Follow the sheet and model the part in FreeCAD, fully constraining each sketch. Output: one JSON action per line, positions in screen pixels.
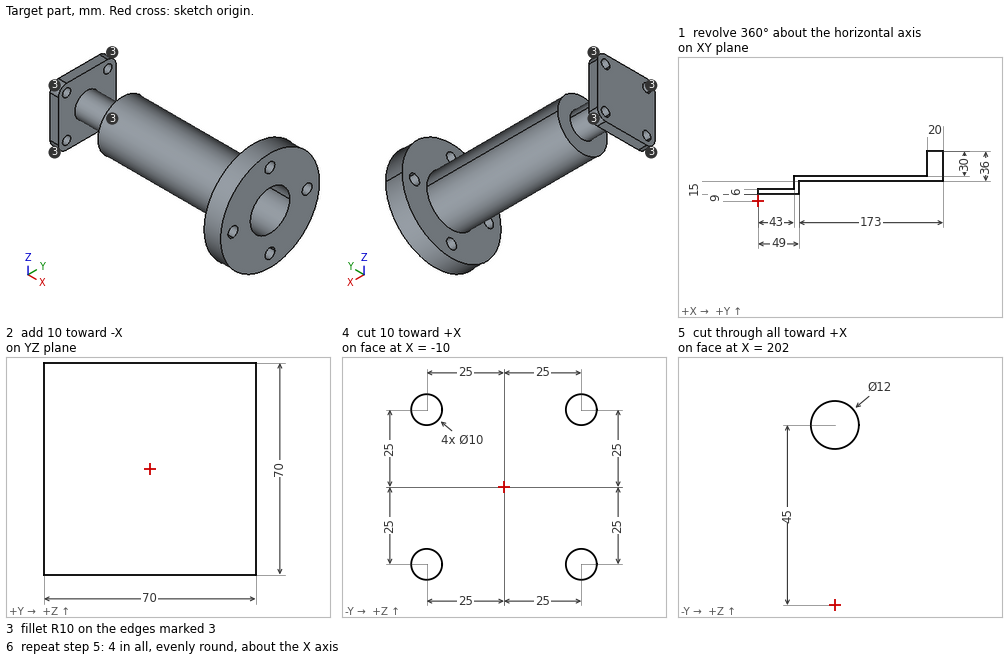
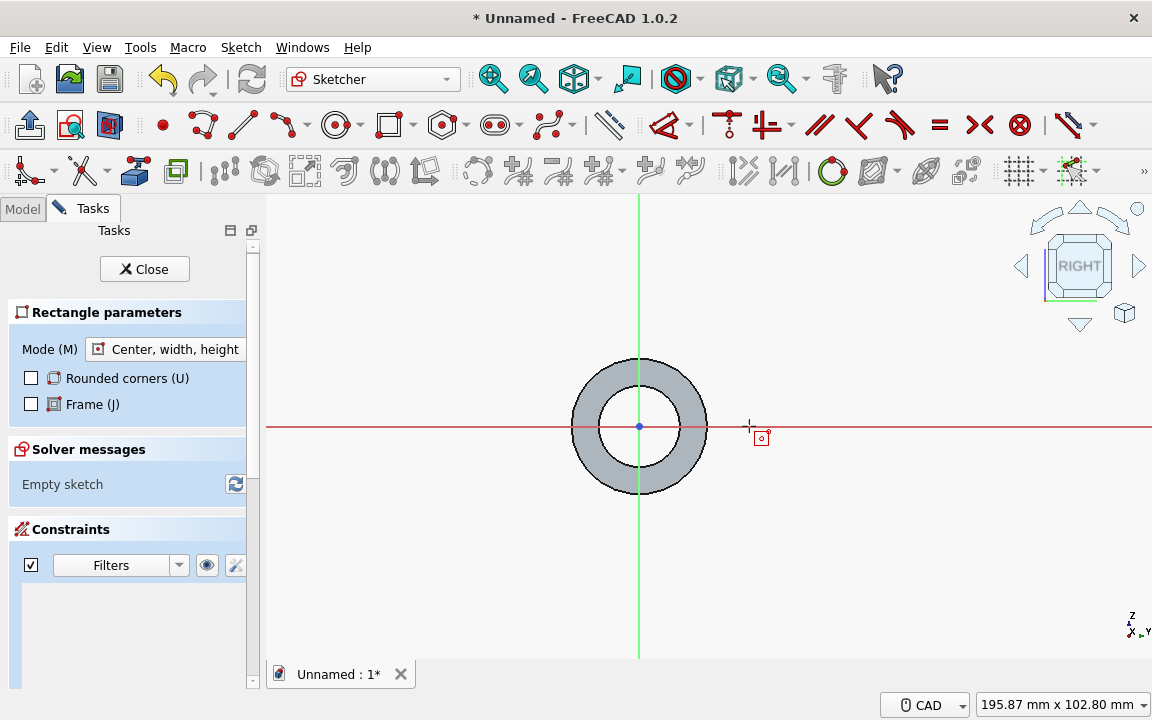
{"action": "left_click", "coordinate": [639, 426]}
{"action": "mouse_move", "coordinate": [798, 268]}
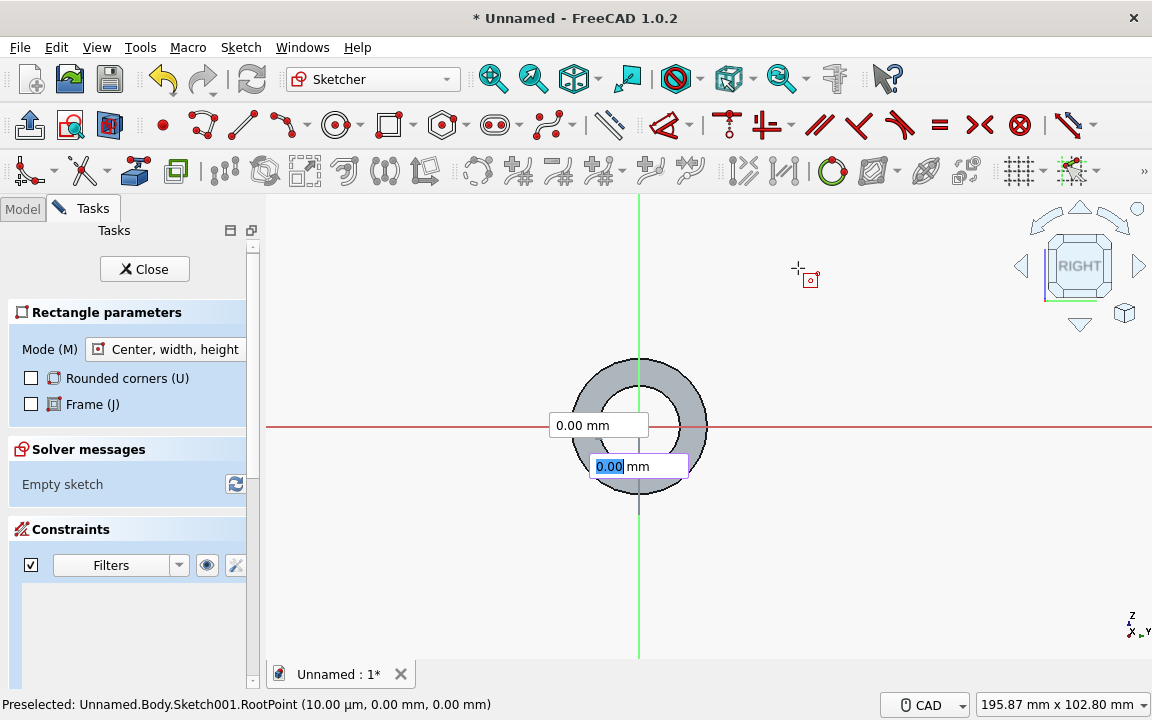
{"action": "type", "text": "70"}
{"action": "key", "text": "Tab"}
{"action": "type", "text": "70"}
{"action": "key", "text": "Return"}
{"action": "key", "text": "Escape"}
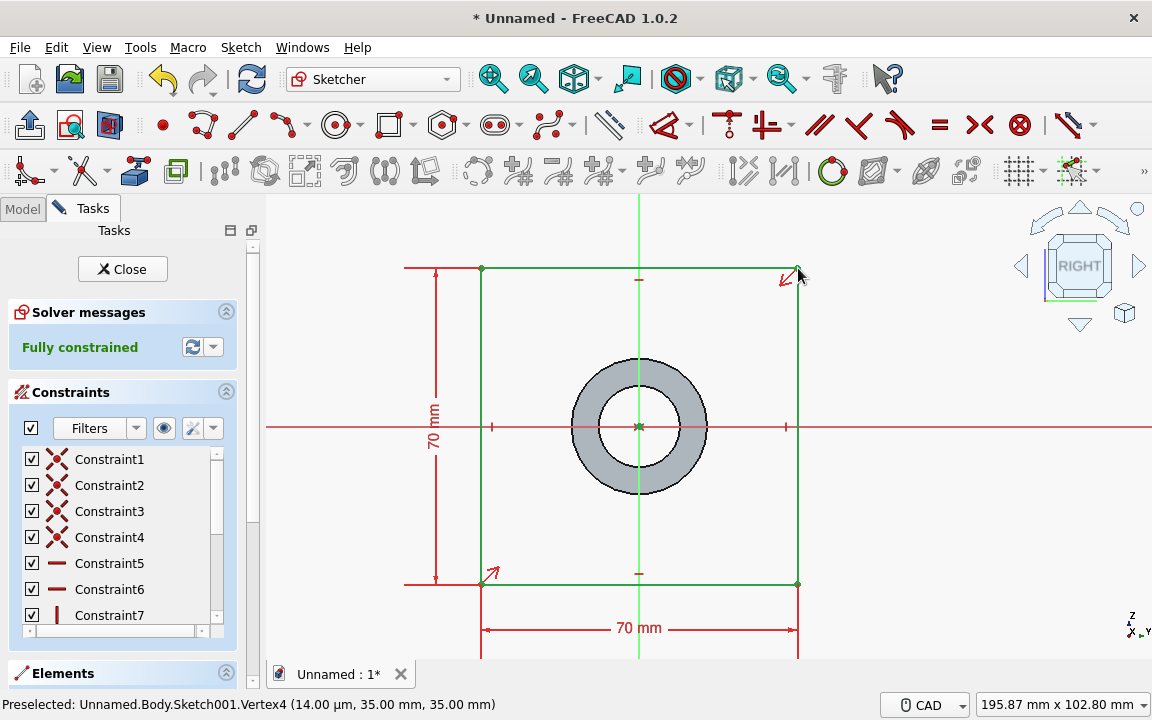
{"action": "left_click", "coordinate": [123, 269]}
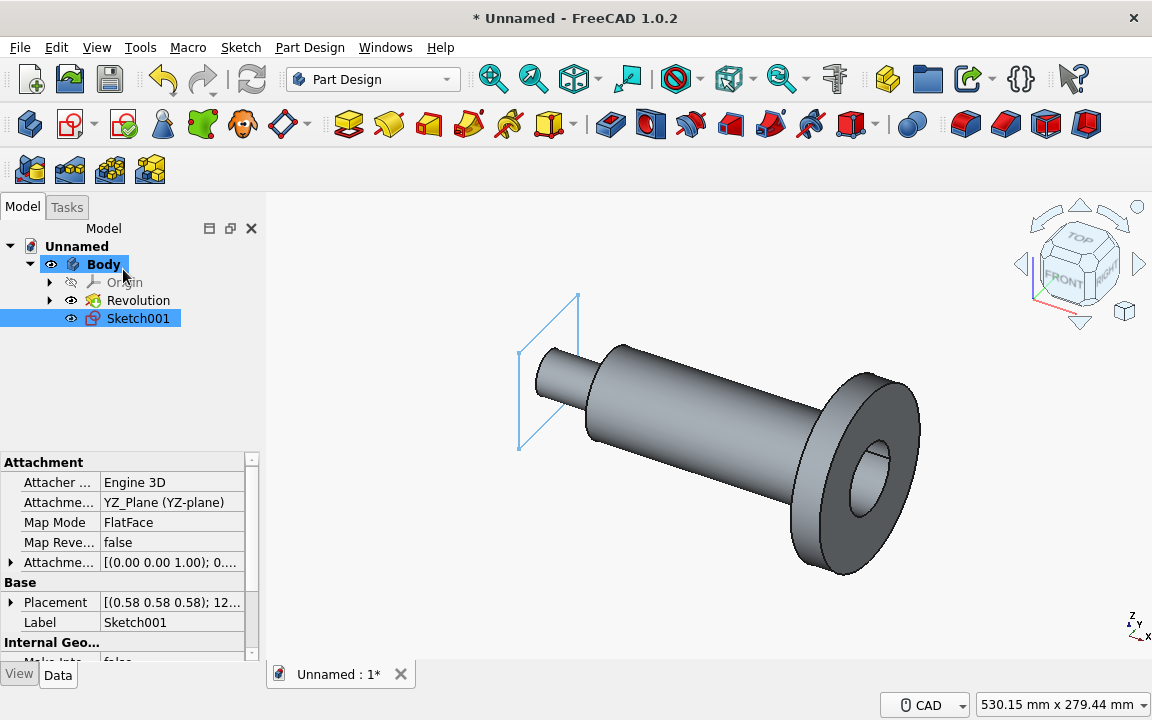
{"action": "left_click", "coordinate": [350, 124]}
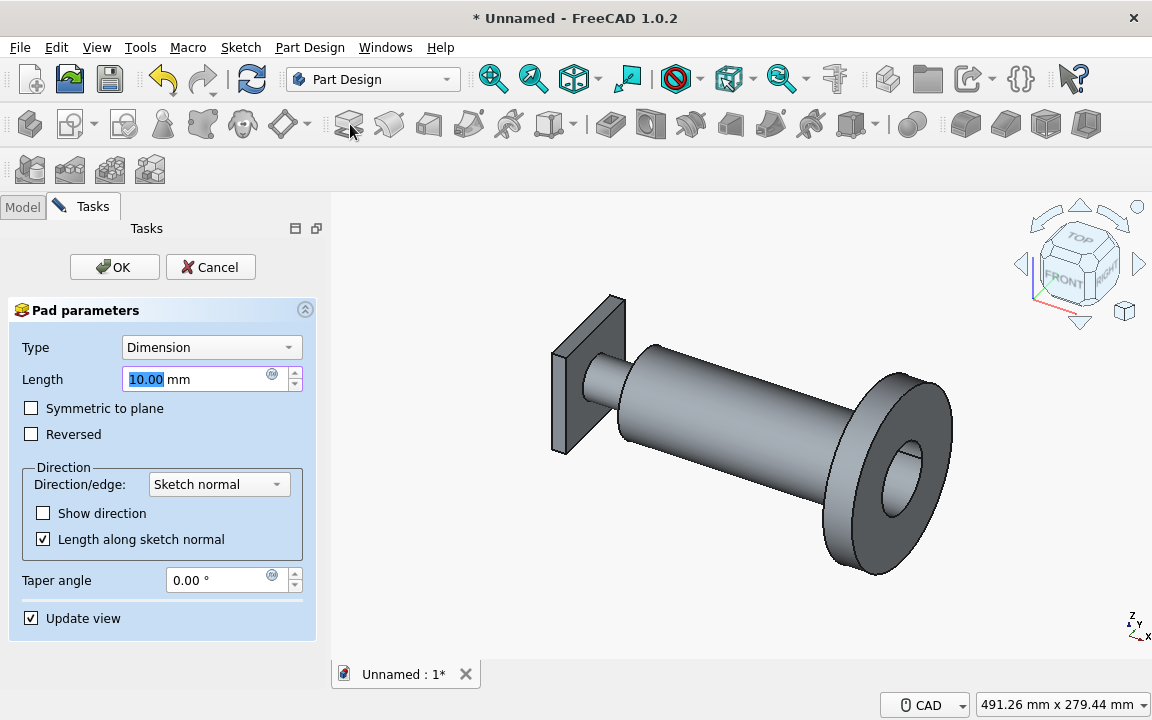
{"action": "type", "text": "10"}
{"action": "key", "text": "Tab"}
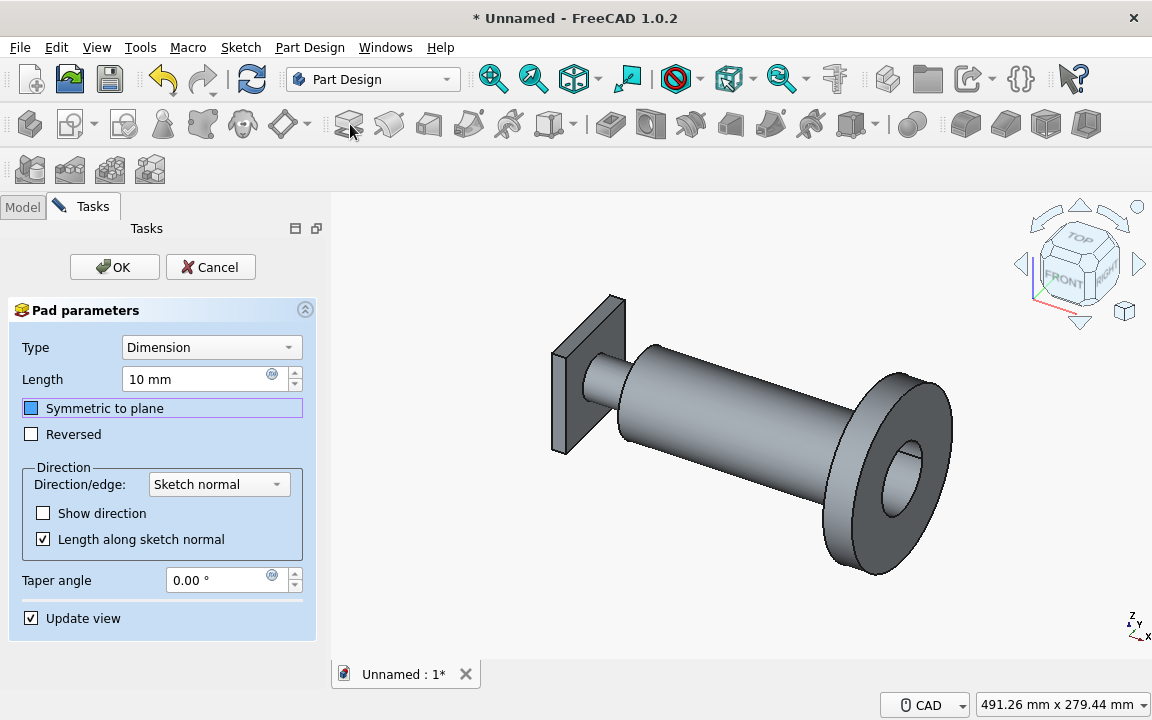
{"action": "left_click", "coordinate": [30, 434]}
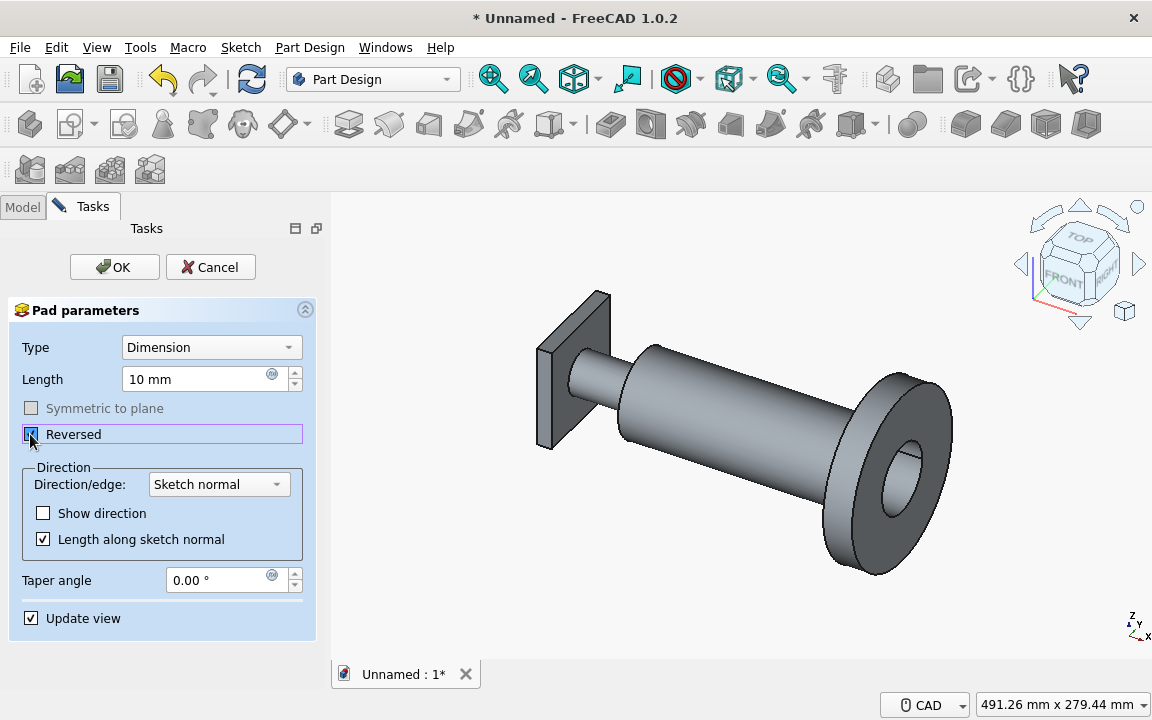
{"action": "left_click", "coordinate": [115, 267]}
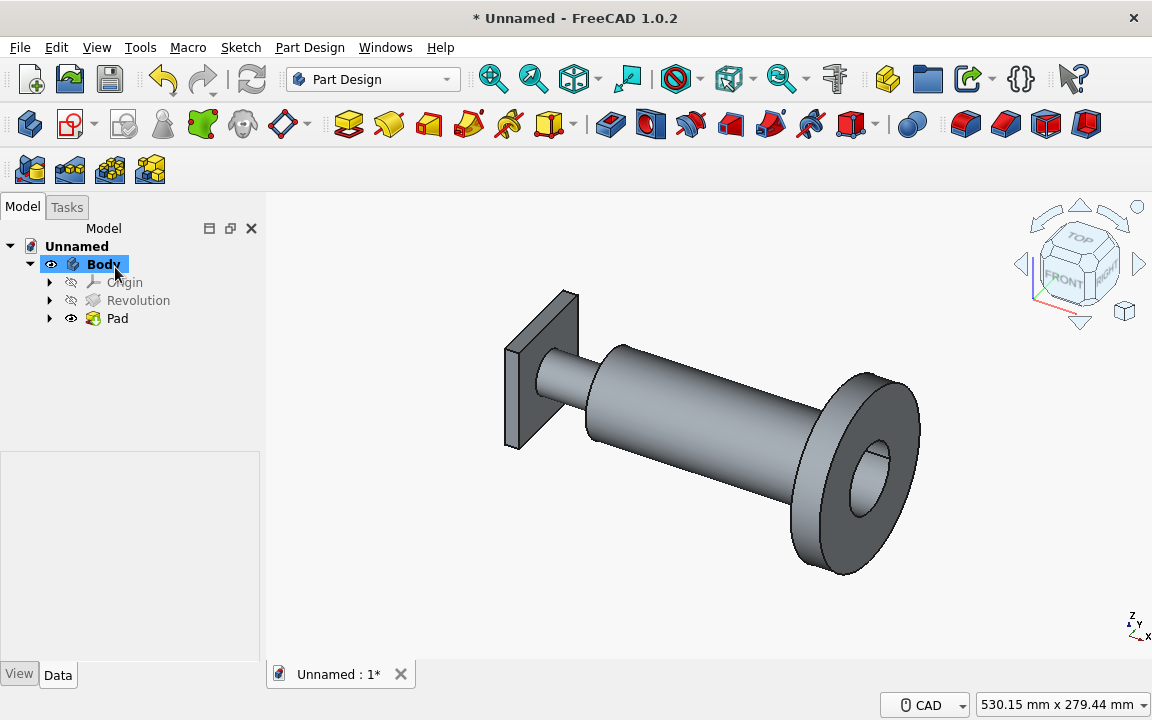
{"action": "left_click", "coordinate": [512, 350]}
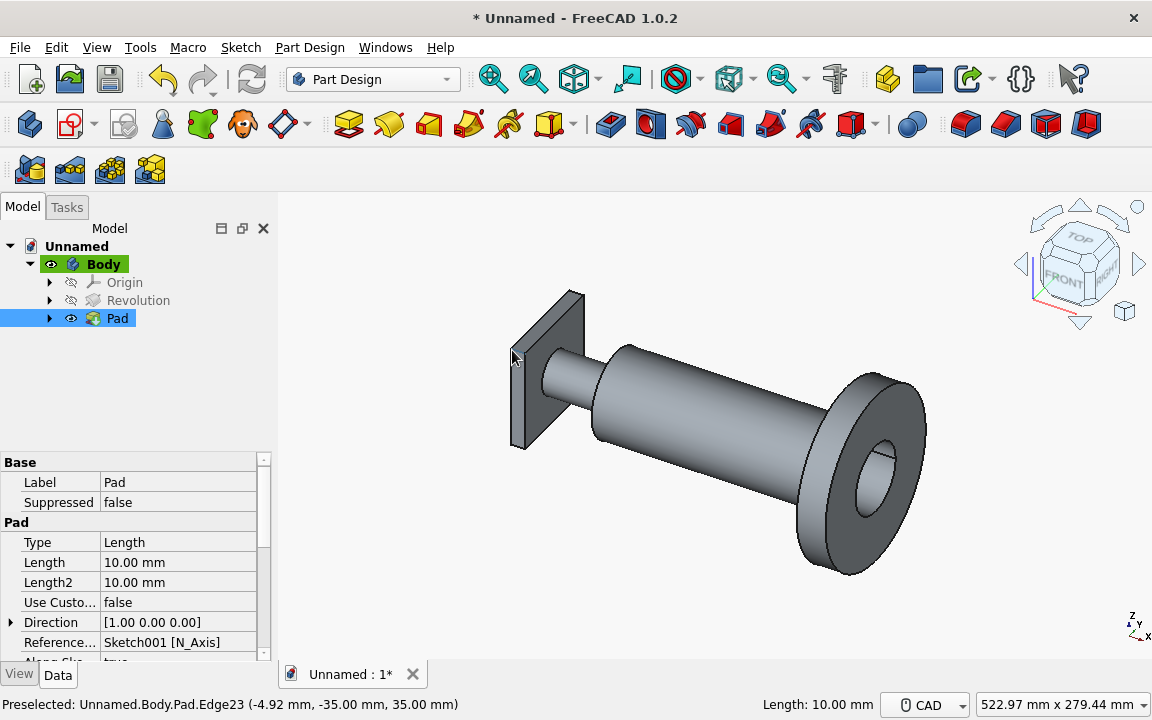
{"action": "scroll", "coordinate": [576, 292], "scroll_direction": "up", "scroll_amount": 5}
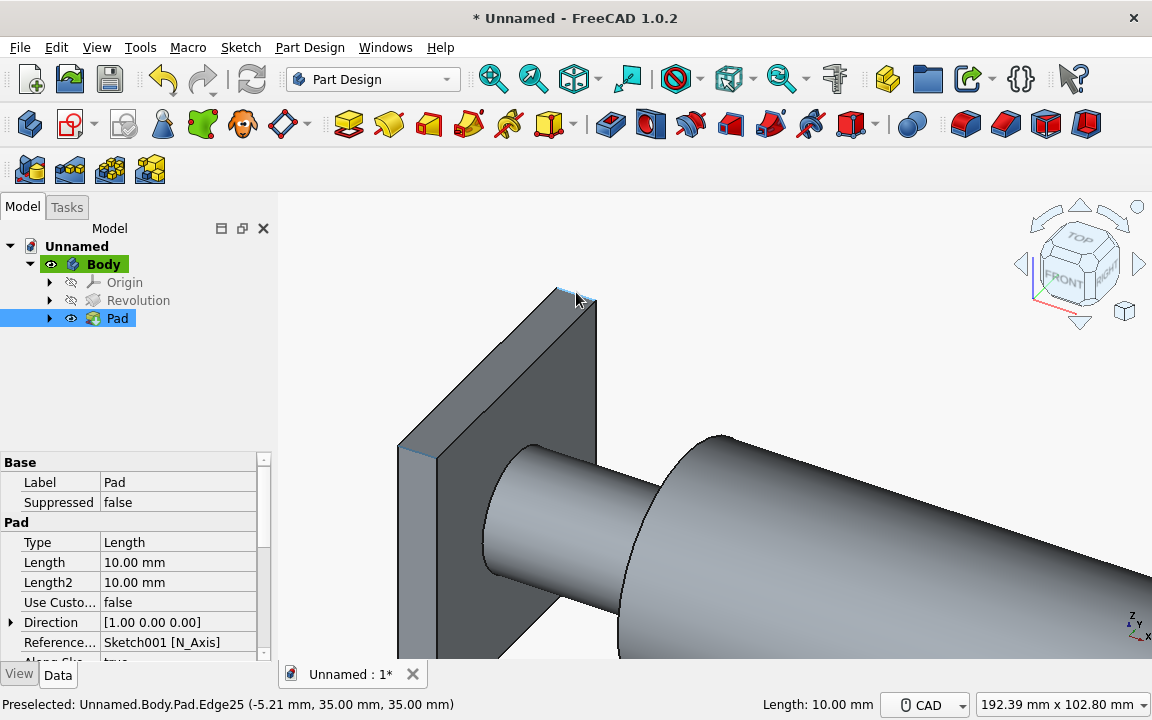
{"action": "left_click", "coordinate": [494, 80]}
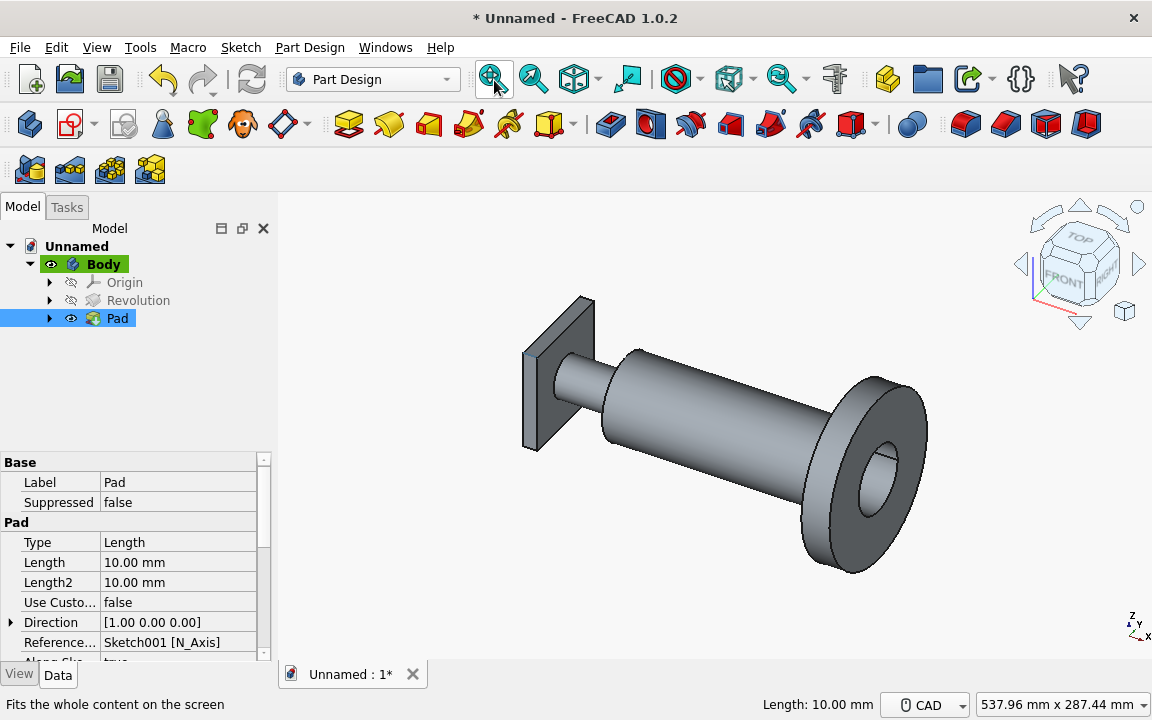
{"action": "key", "text": "0"}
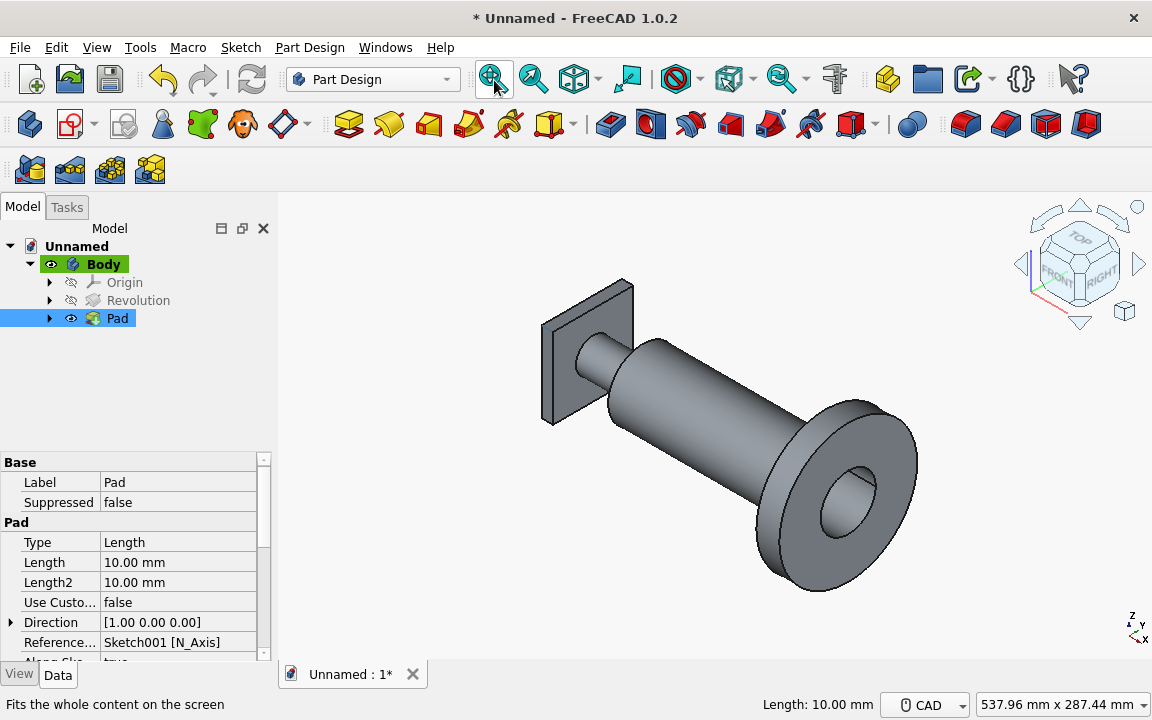
{"action": "scroll", "coordinate": [628, 281], "scroll_direction": "up", "scroll_amount": 5}